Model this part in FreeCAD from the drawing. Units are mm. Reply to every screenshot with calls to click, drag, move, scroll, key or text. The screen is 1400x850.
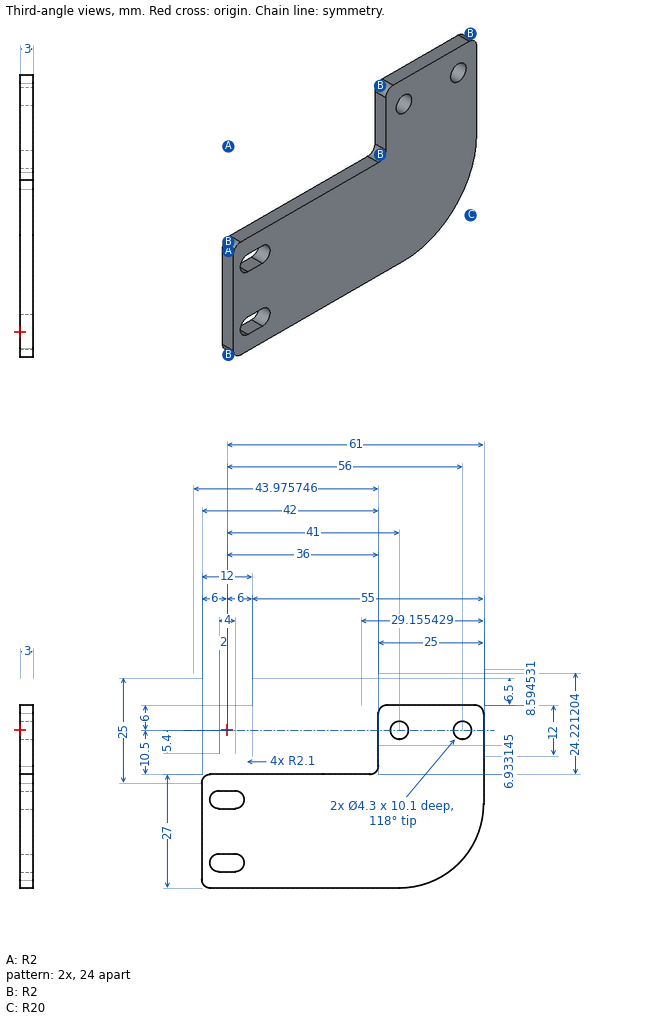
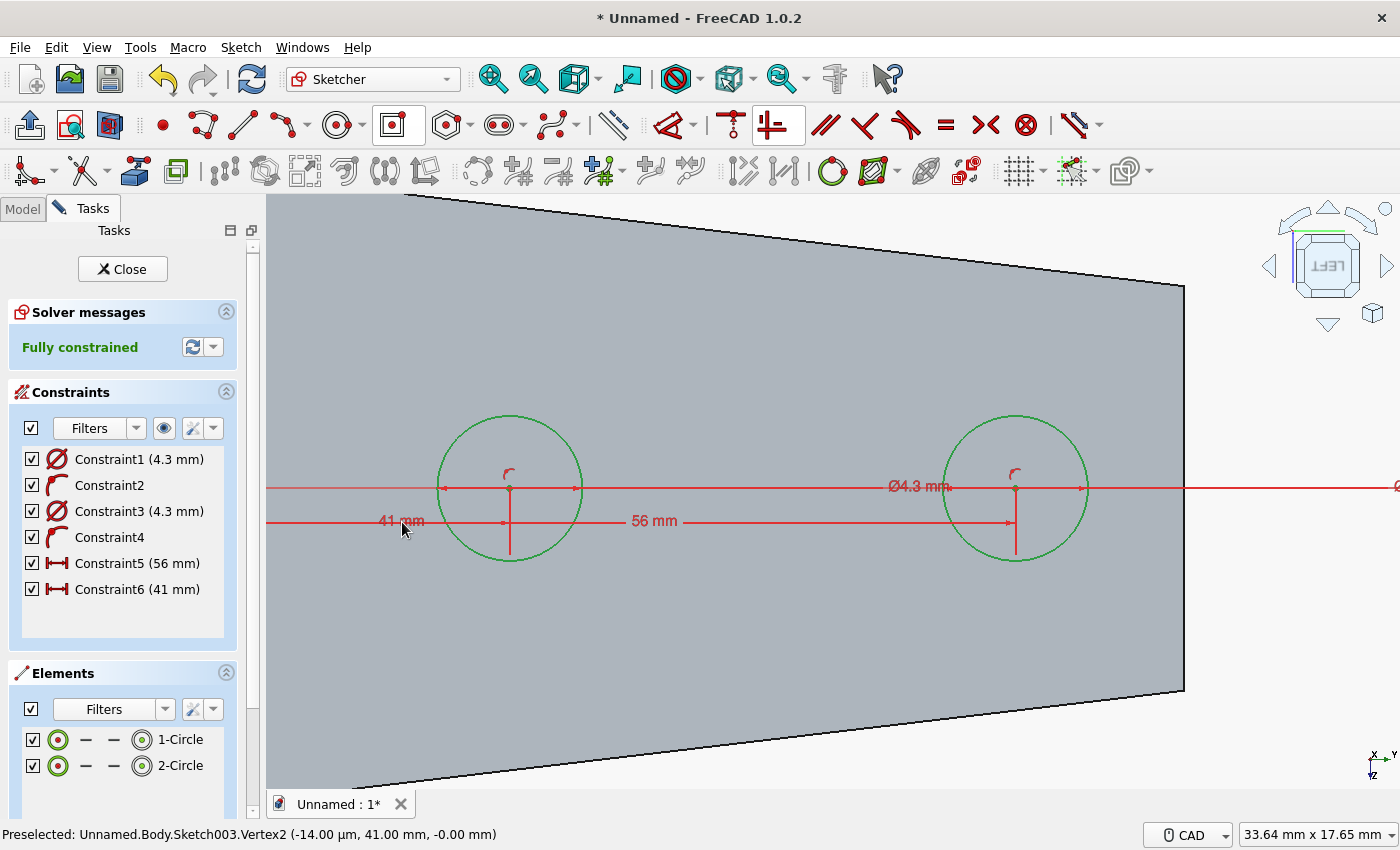
click(123, 269)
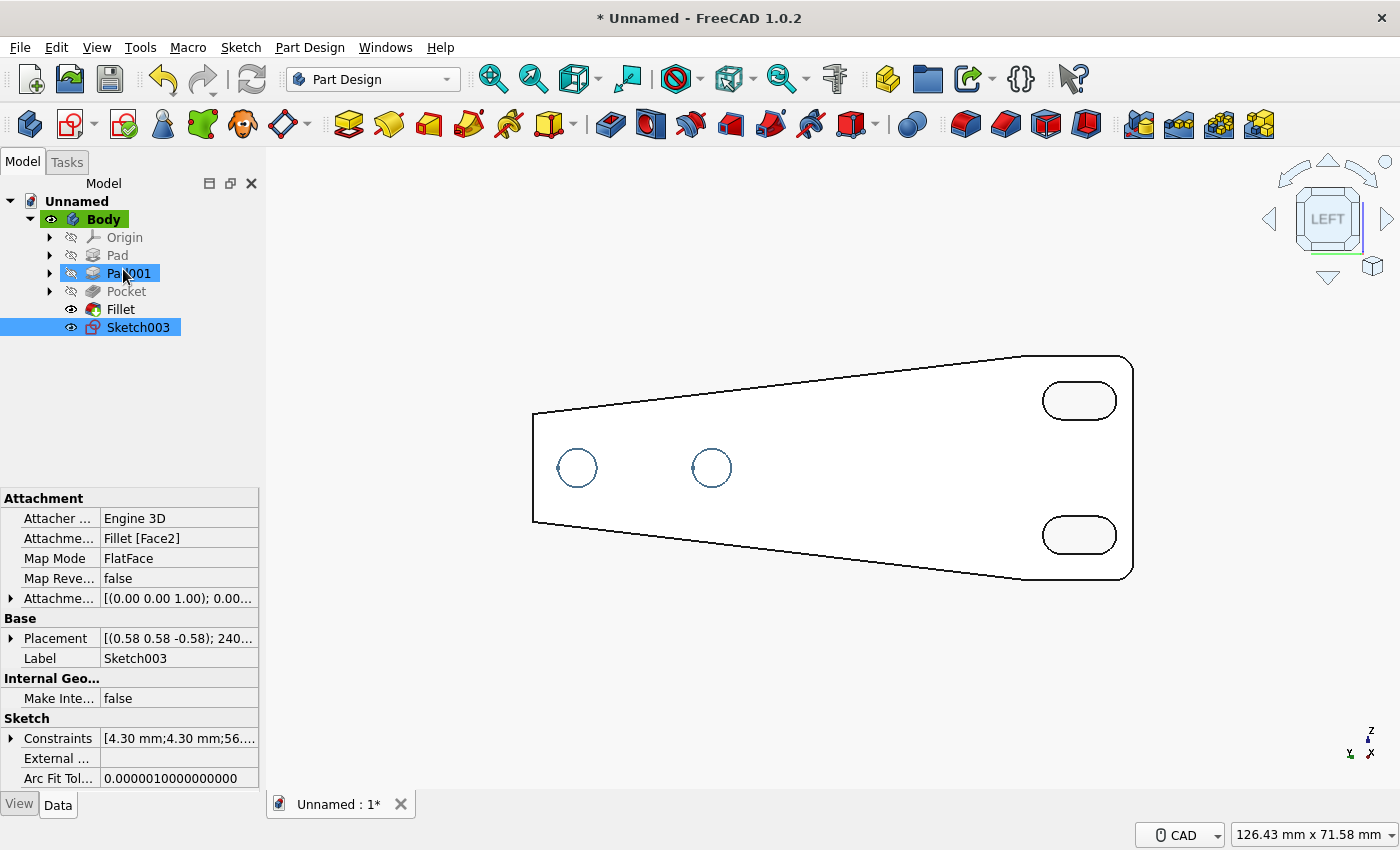
click(652, 124)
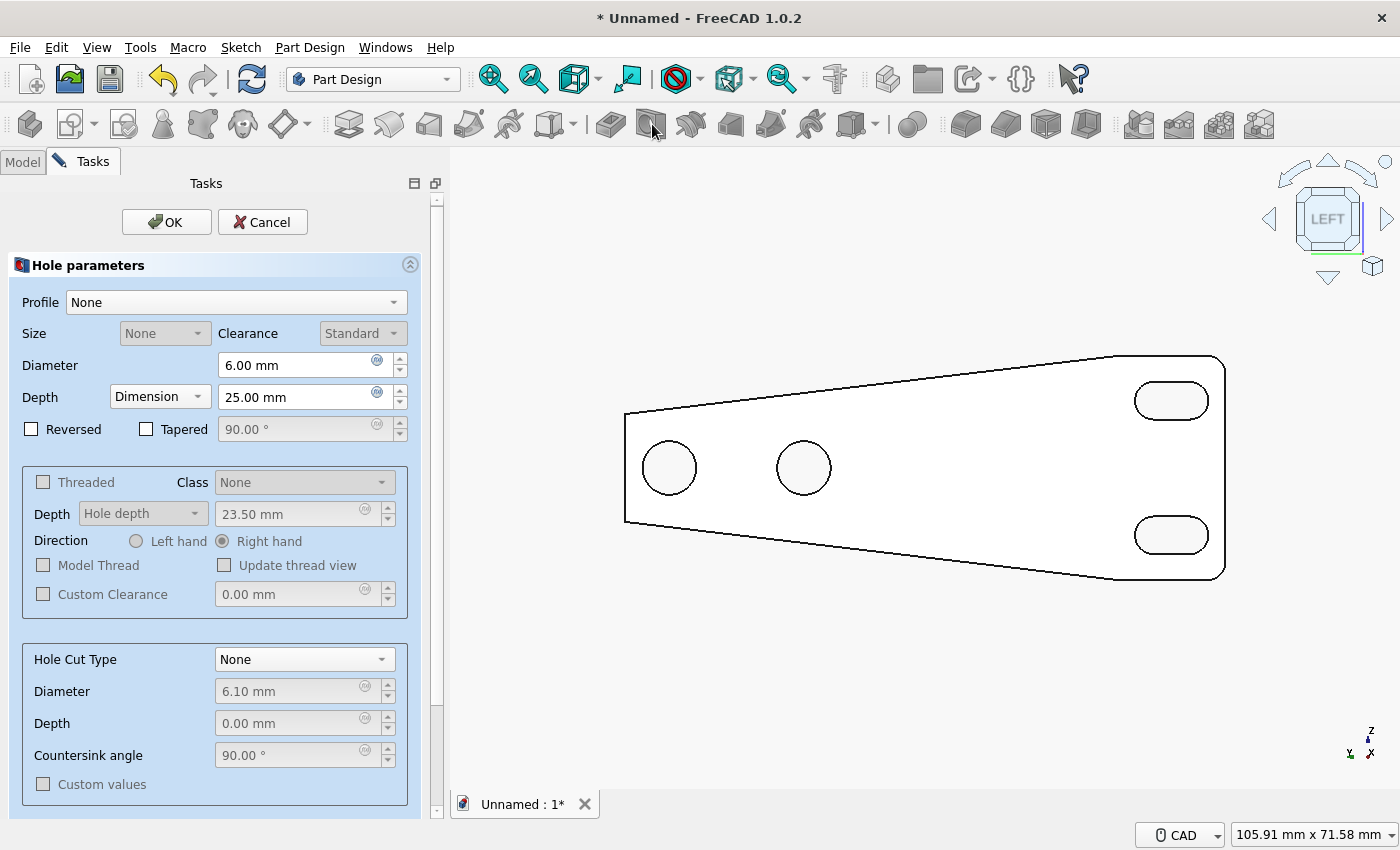
triple_click(305, 365)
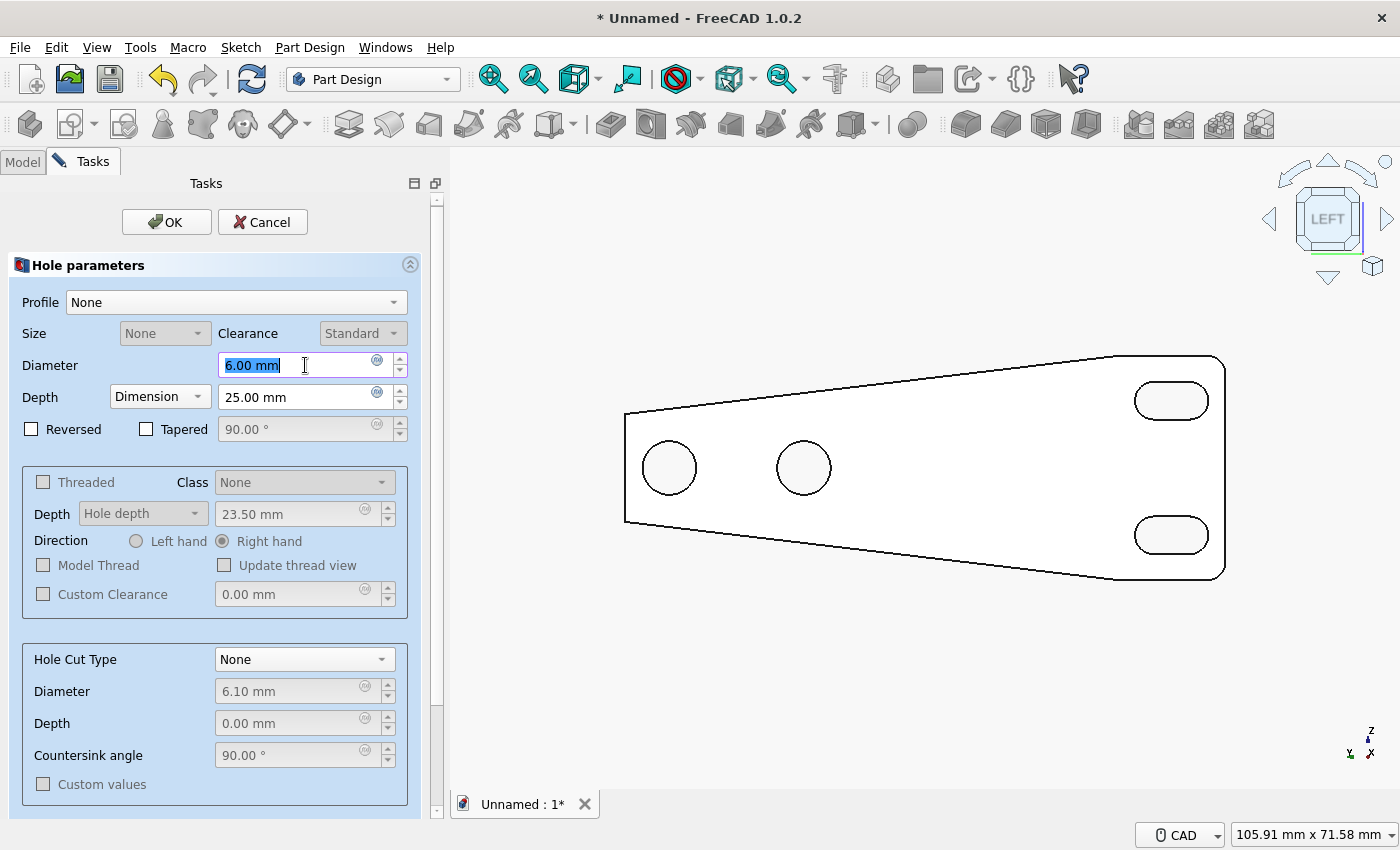
text(4.3)
key(Tab)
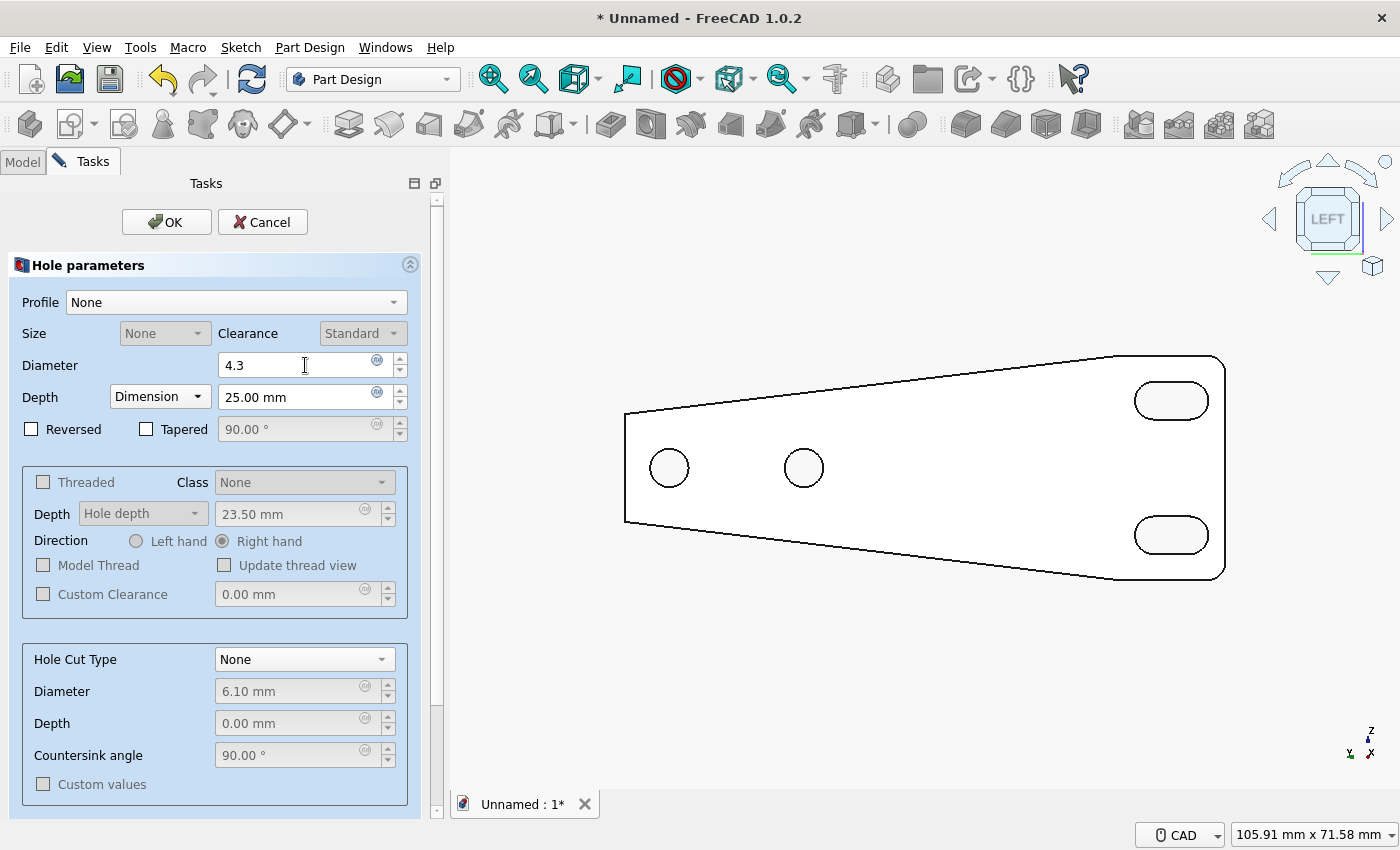
triple_click(305, 397)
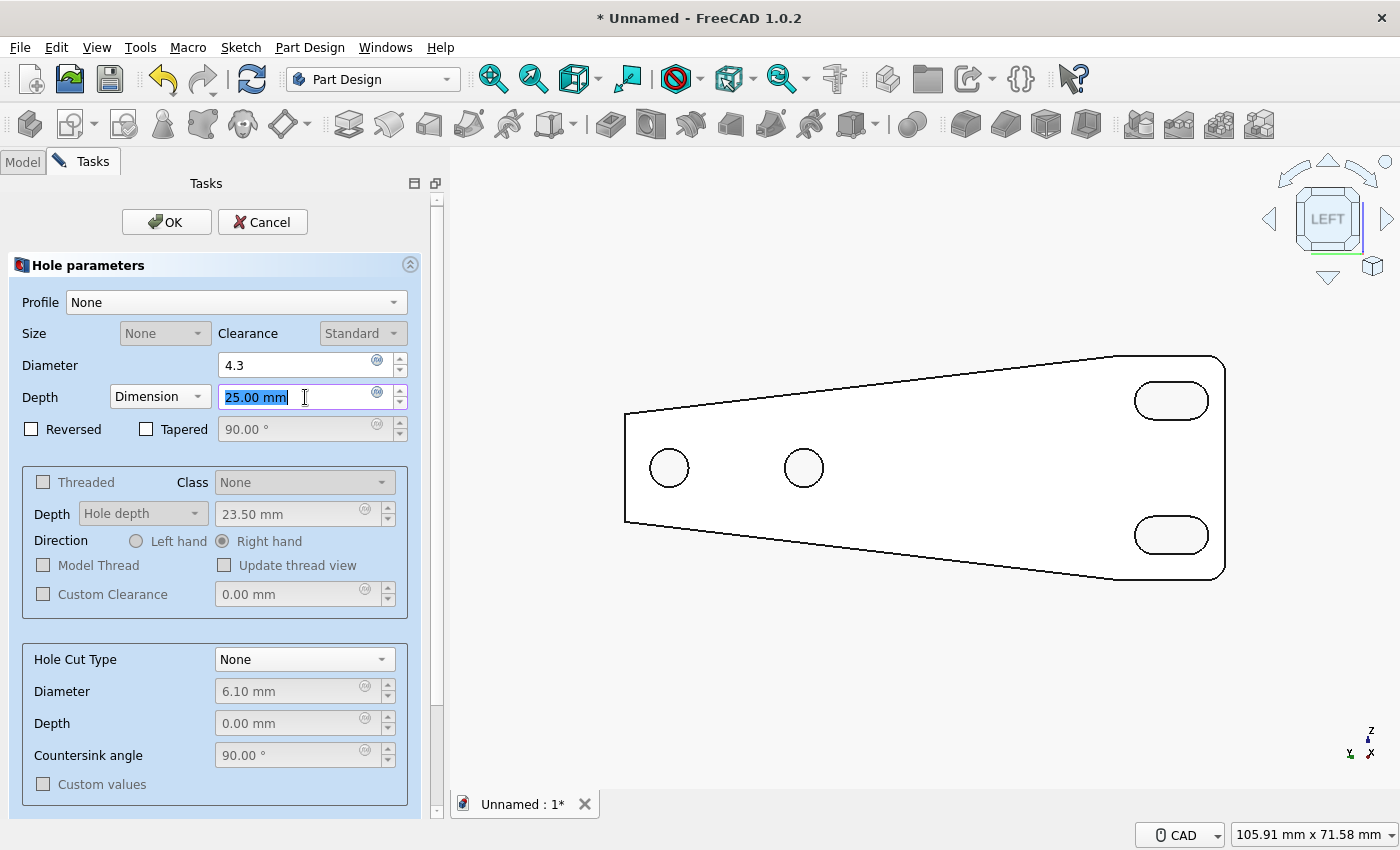
text(10.1)
key(Tab)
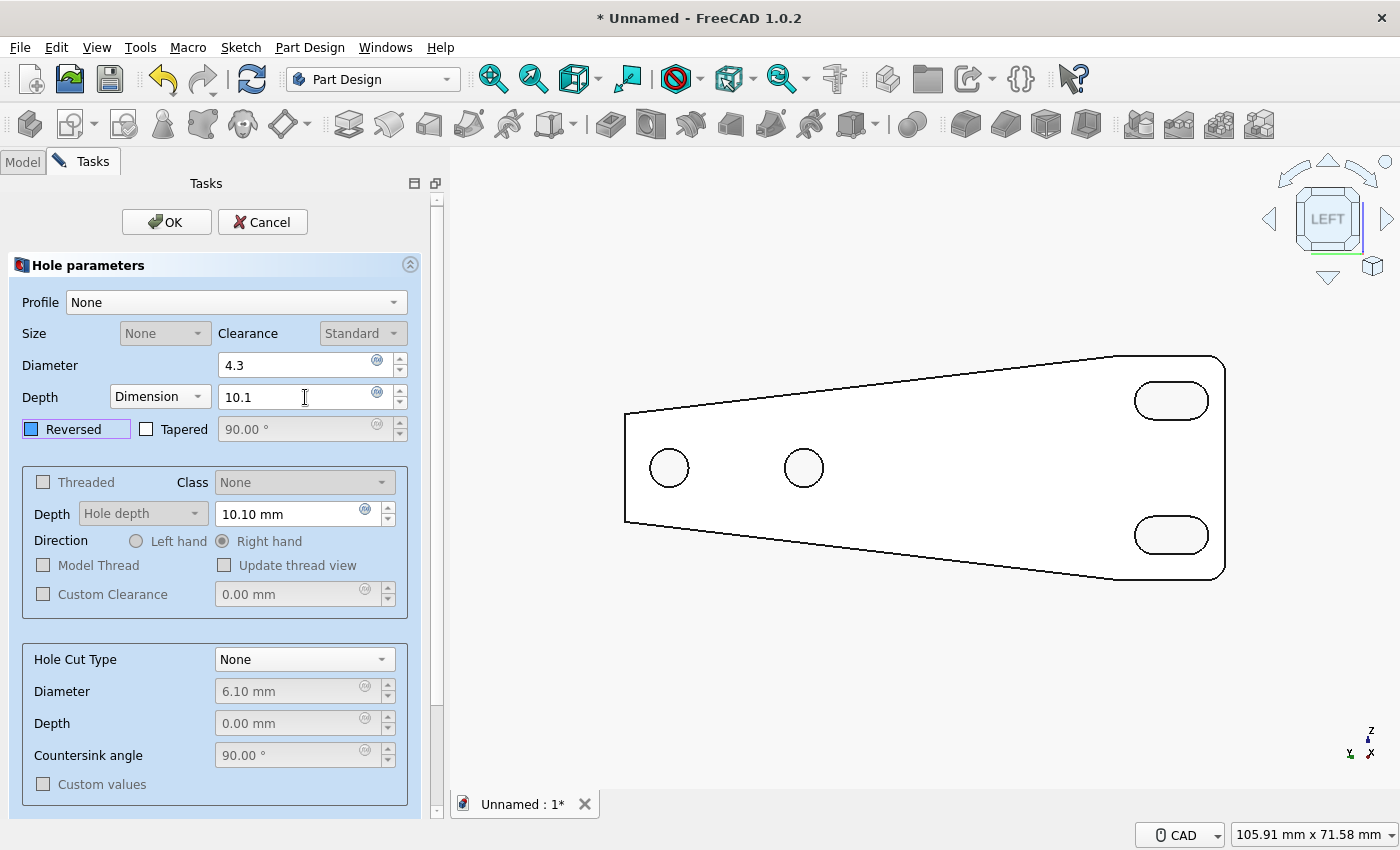
click(167, 222)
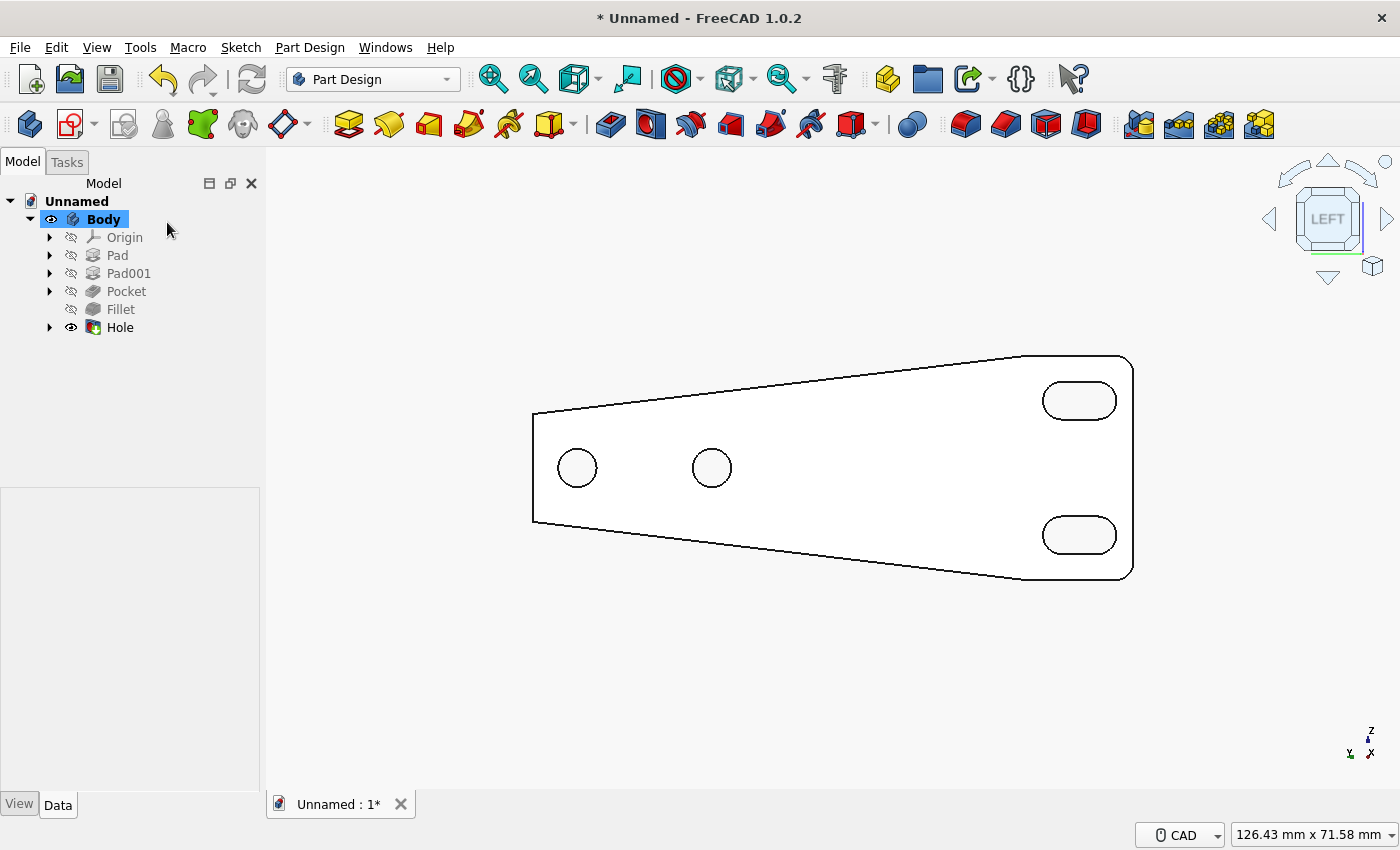
click(919, 467)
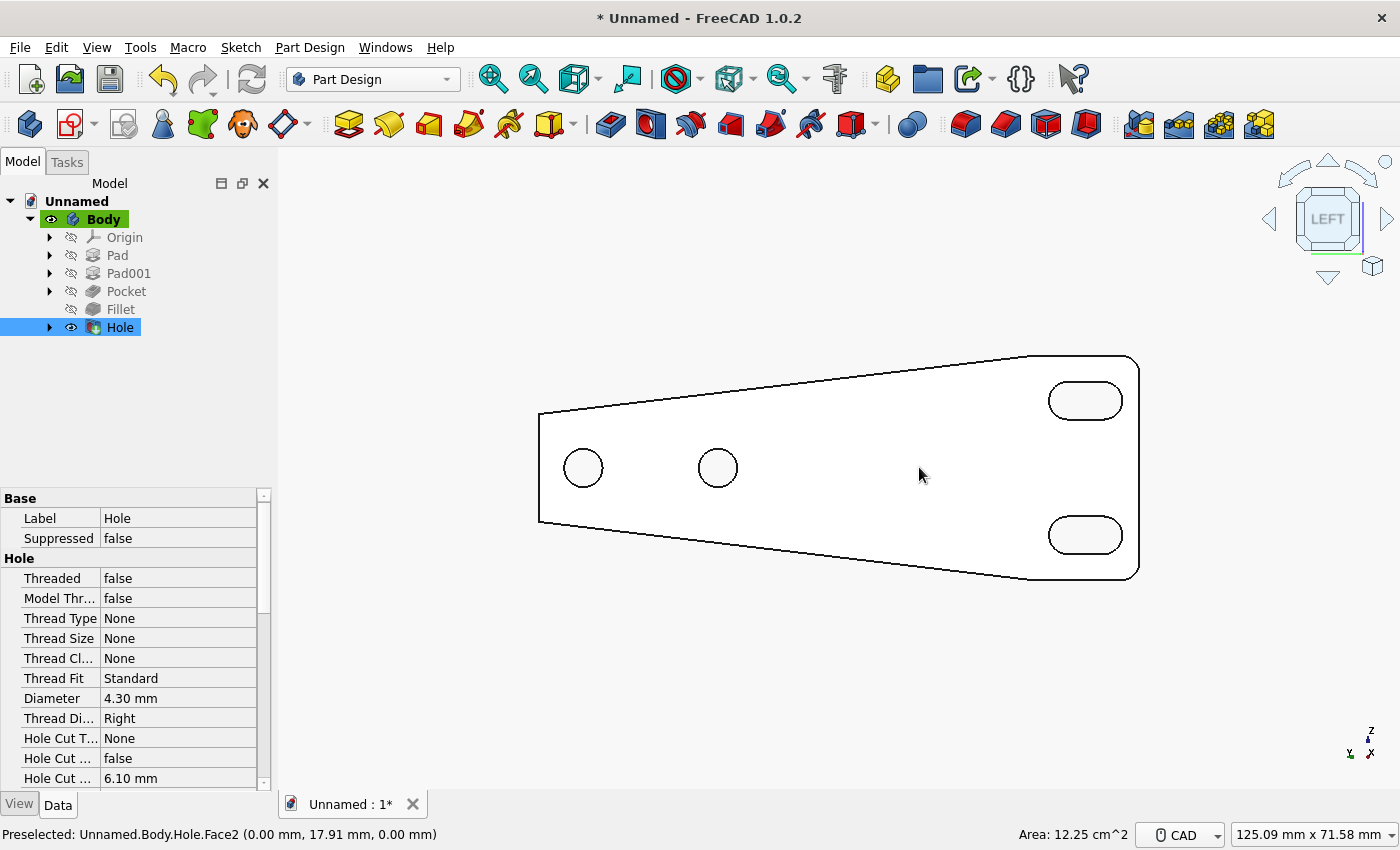
click(70, 124)